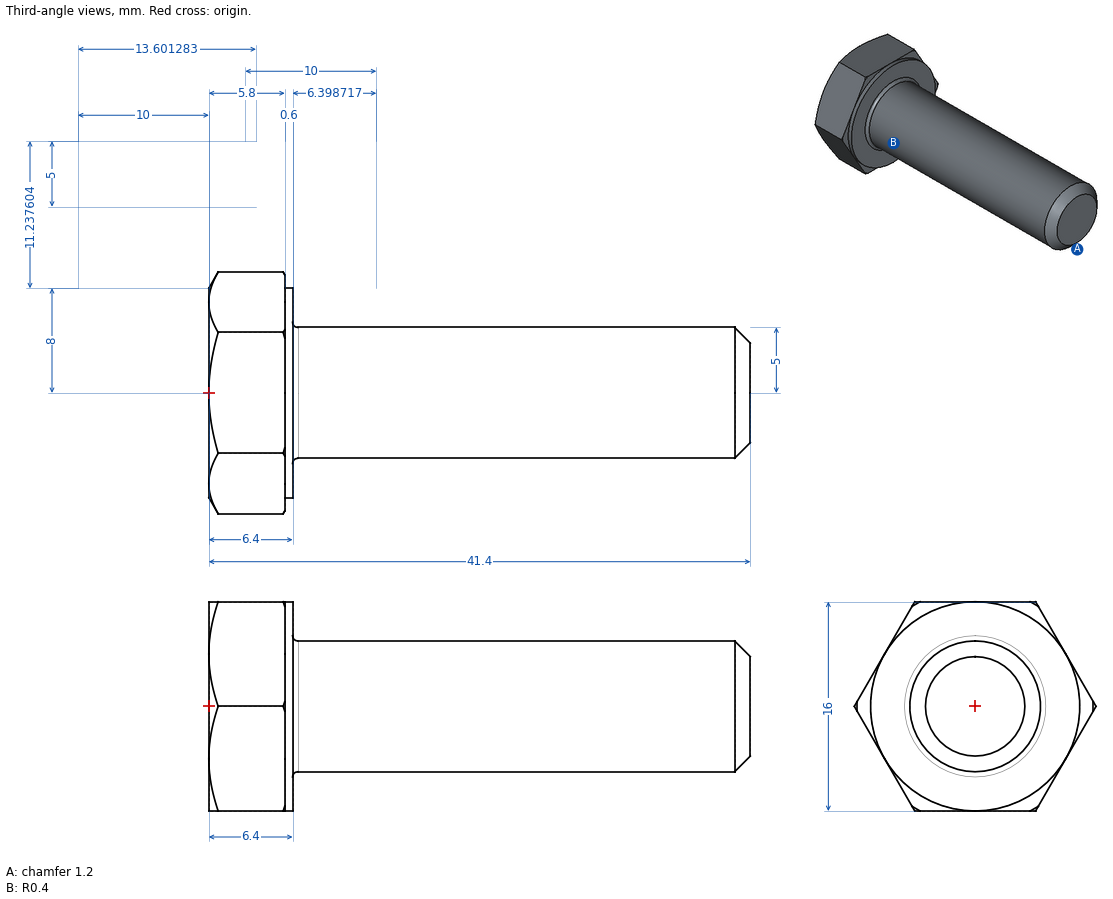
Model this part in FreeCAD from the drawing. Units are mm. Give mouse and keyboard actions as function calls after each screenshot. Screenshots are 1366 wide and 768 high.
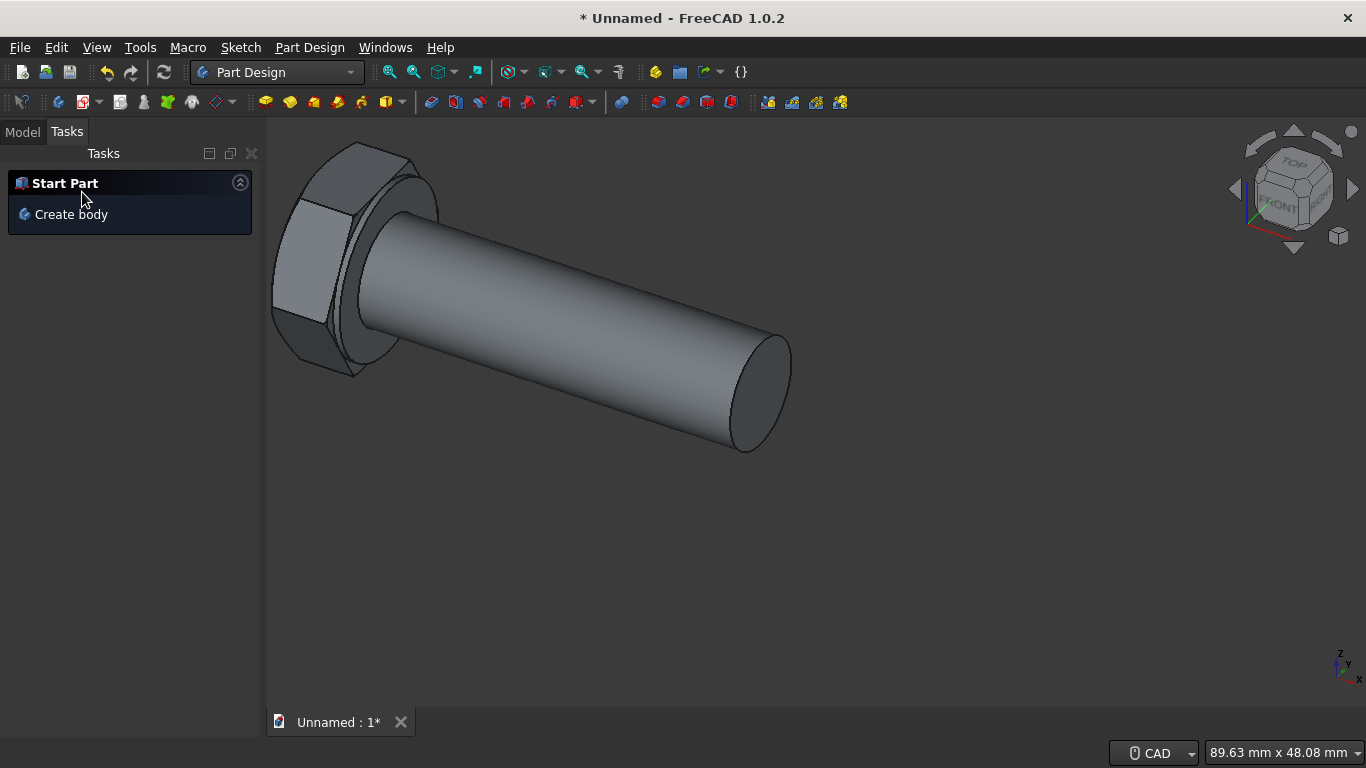
click(390, 72)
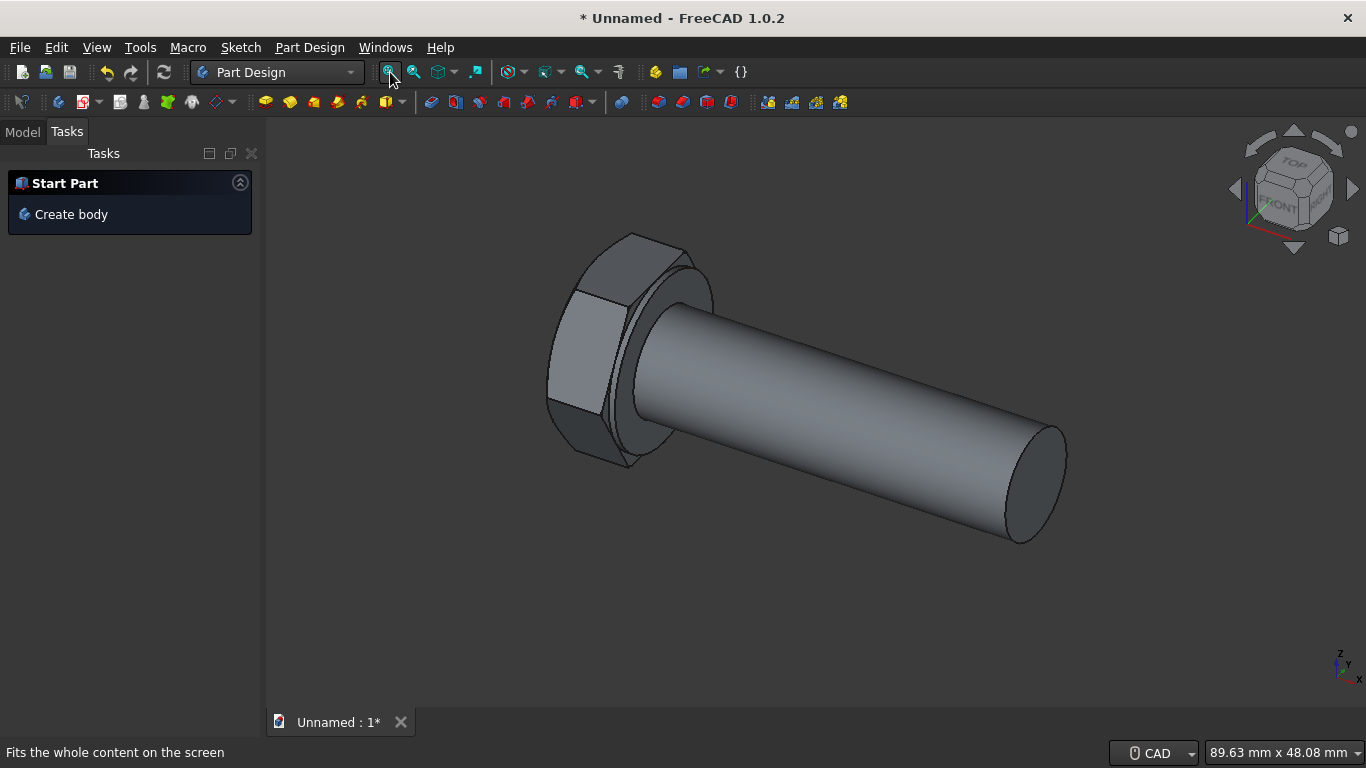
click(1005, 514)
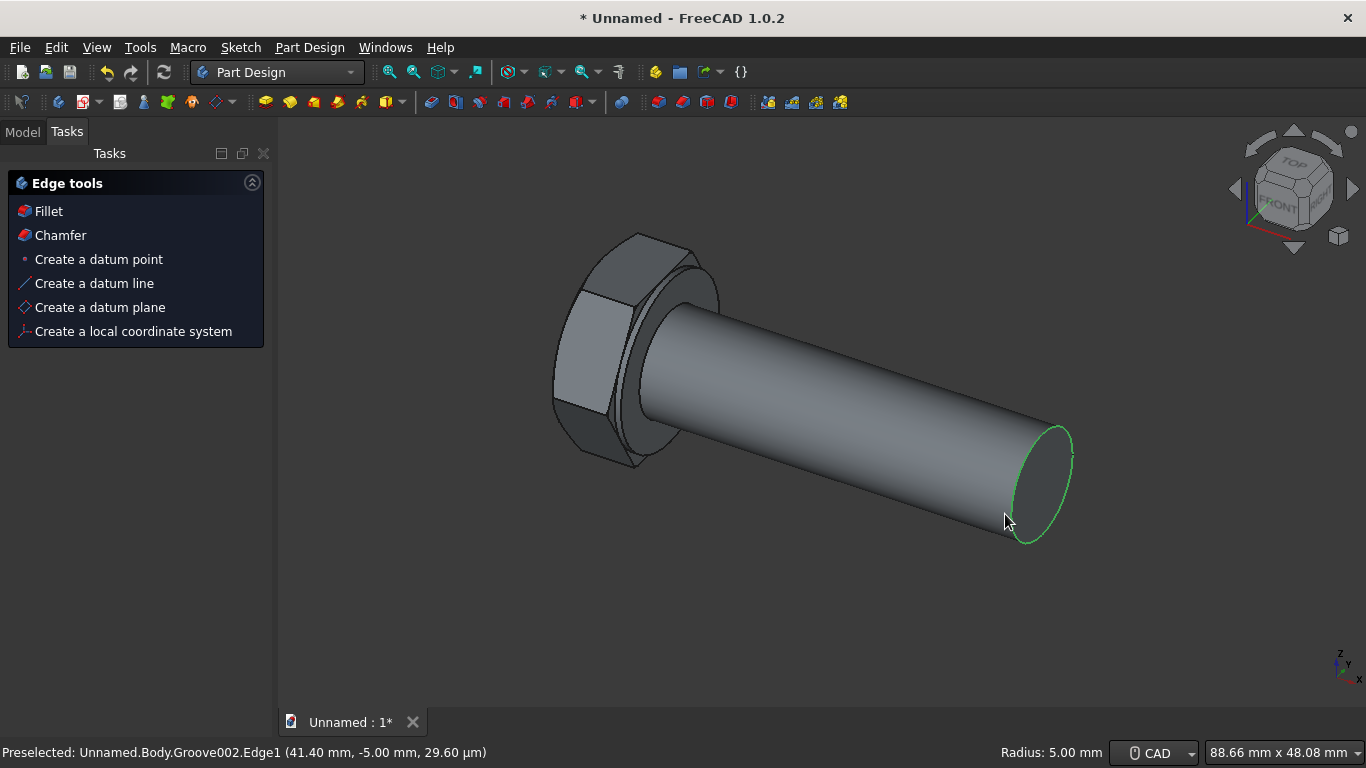
click(684, 102)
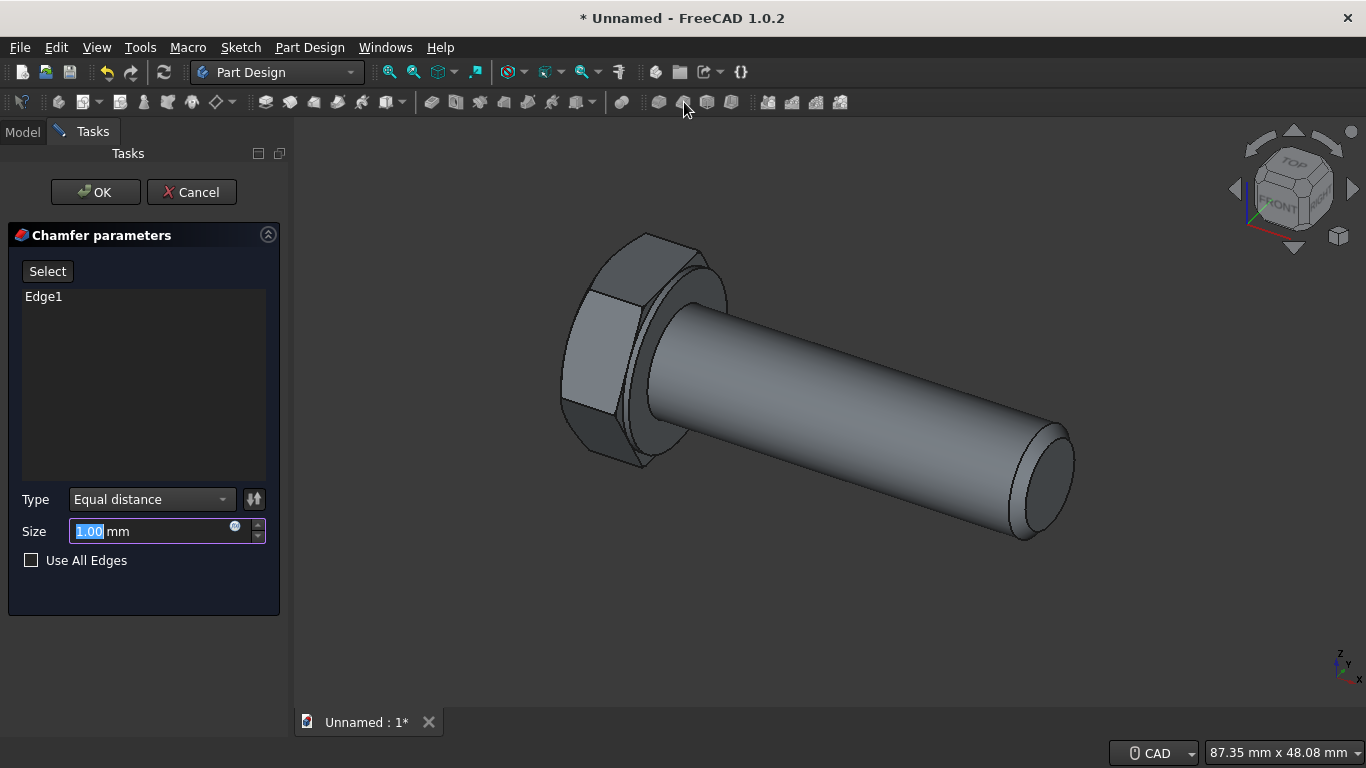
text(1.2)
key(Tab)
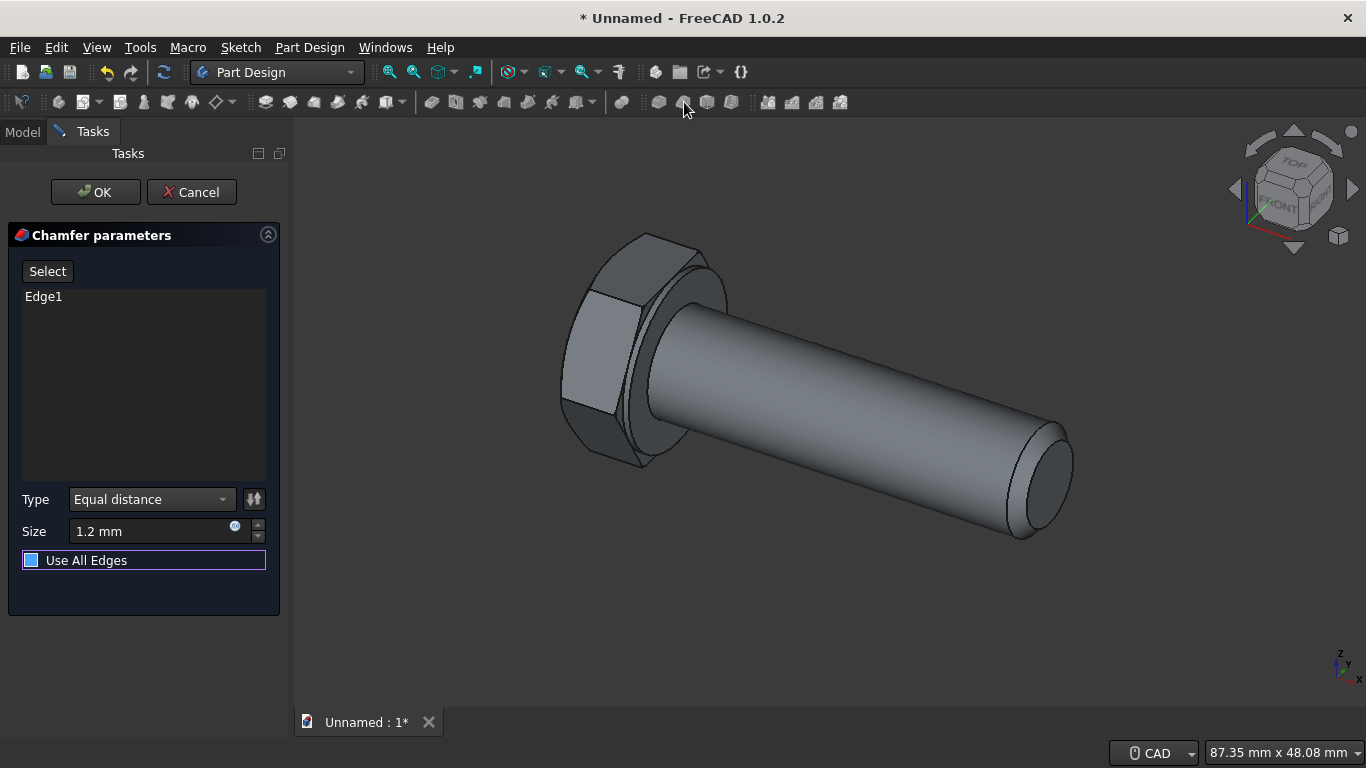
click(96, 192)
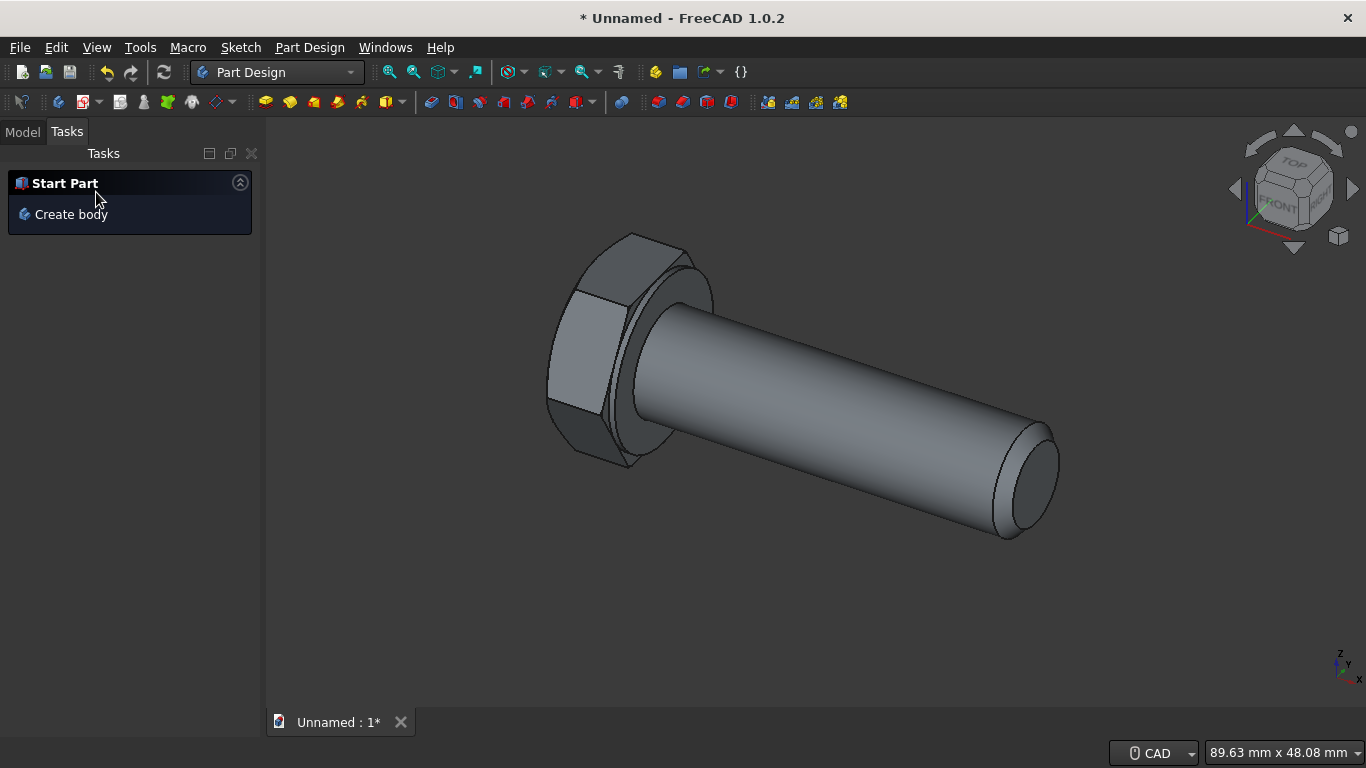
key(0)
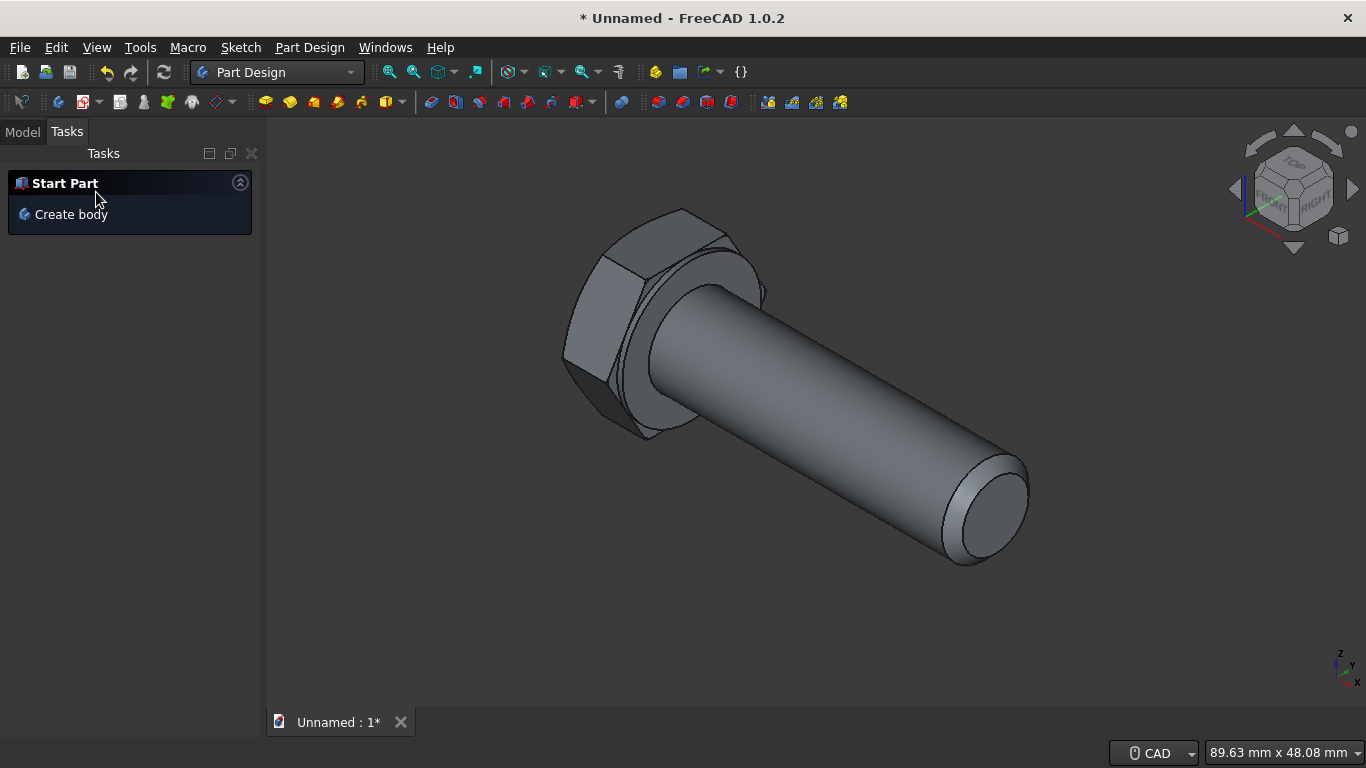
key(2)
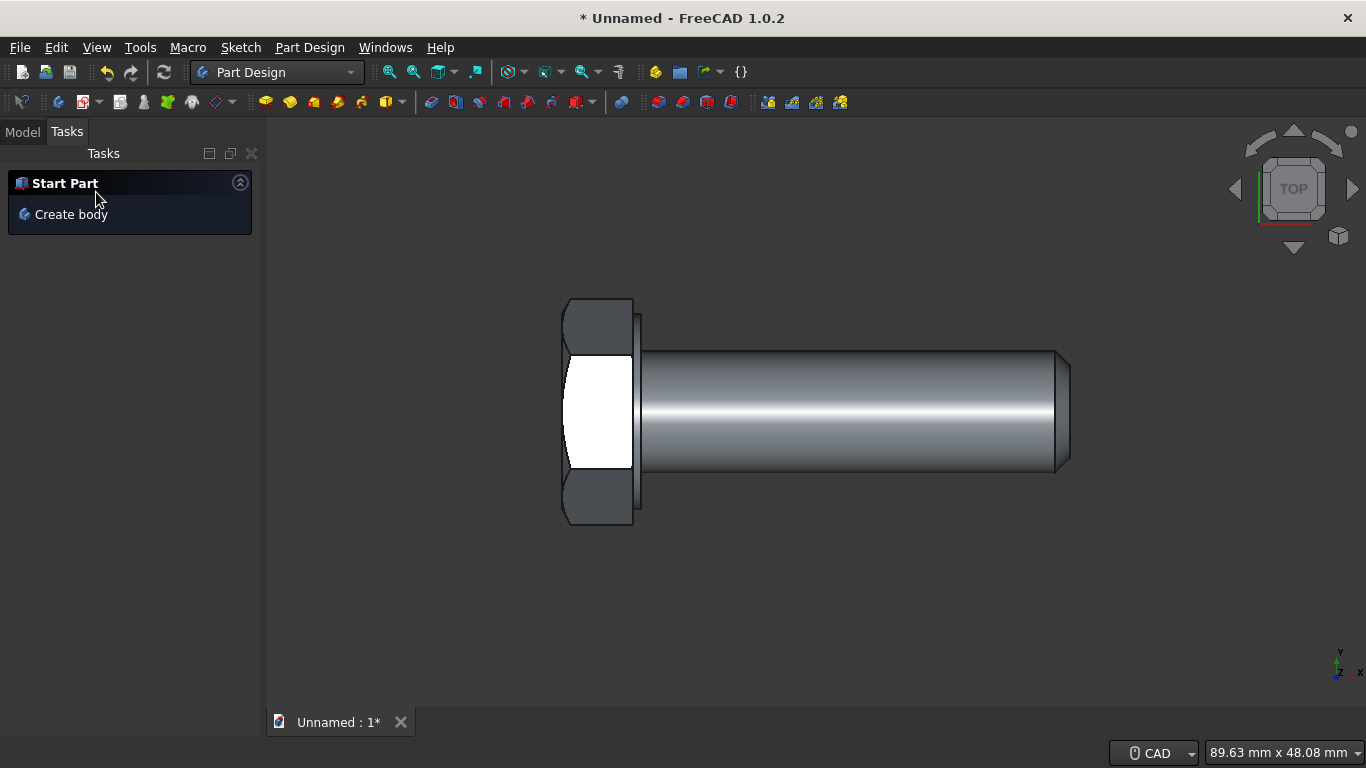
key(1)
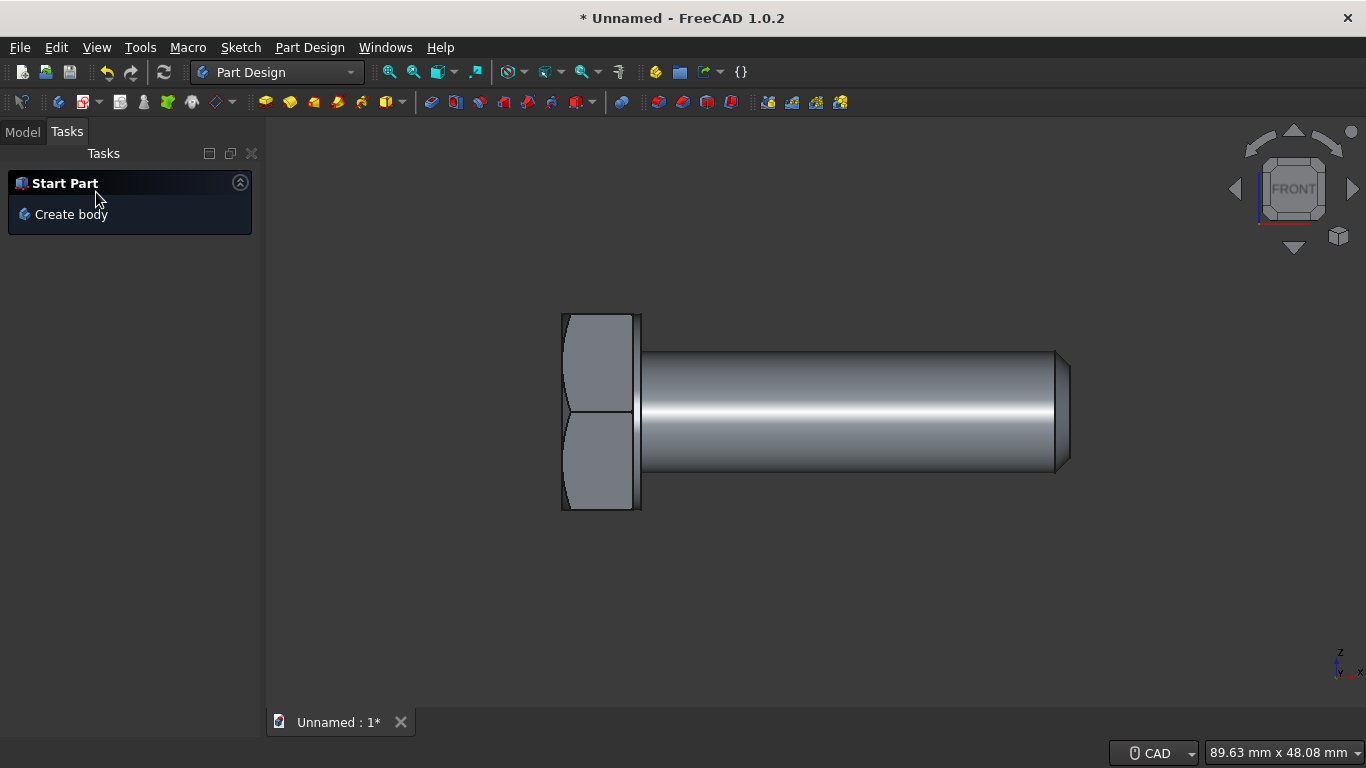
key(3)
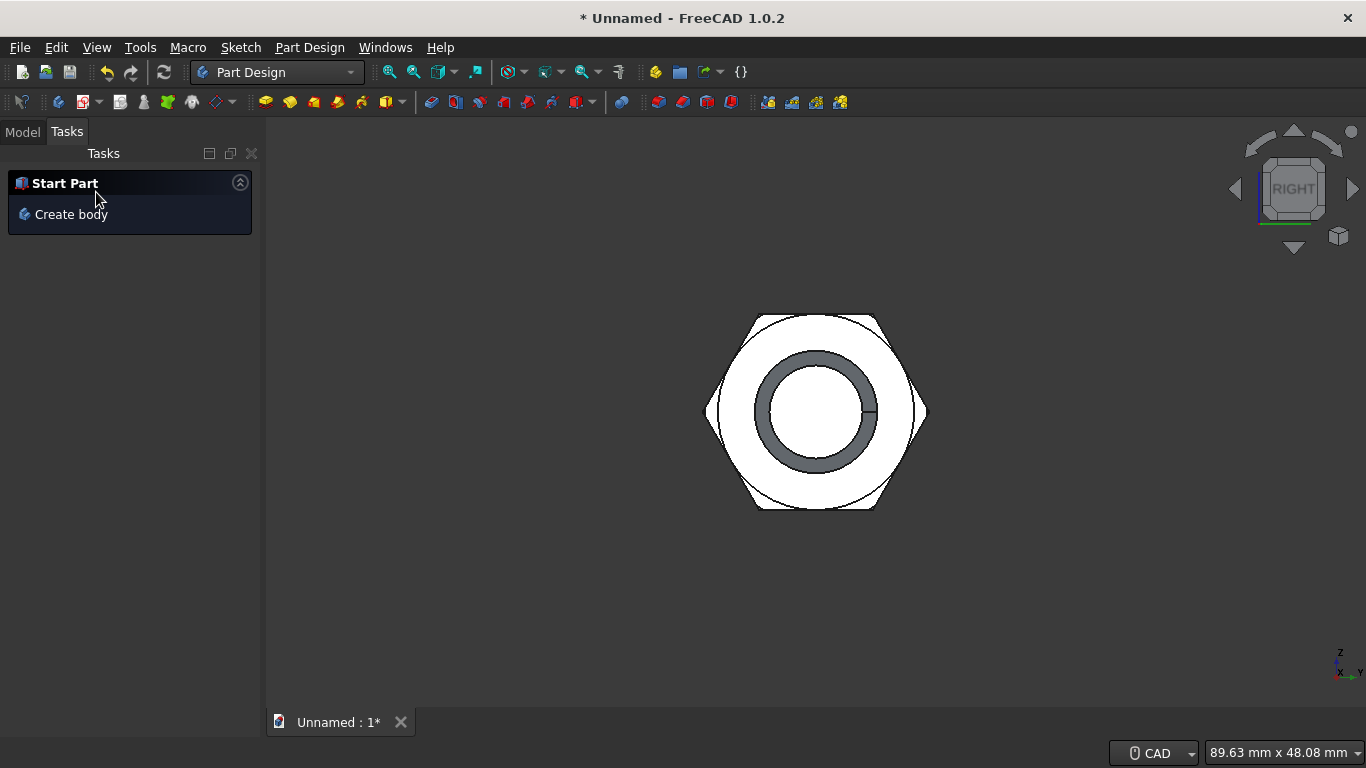
click(390, 72)